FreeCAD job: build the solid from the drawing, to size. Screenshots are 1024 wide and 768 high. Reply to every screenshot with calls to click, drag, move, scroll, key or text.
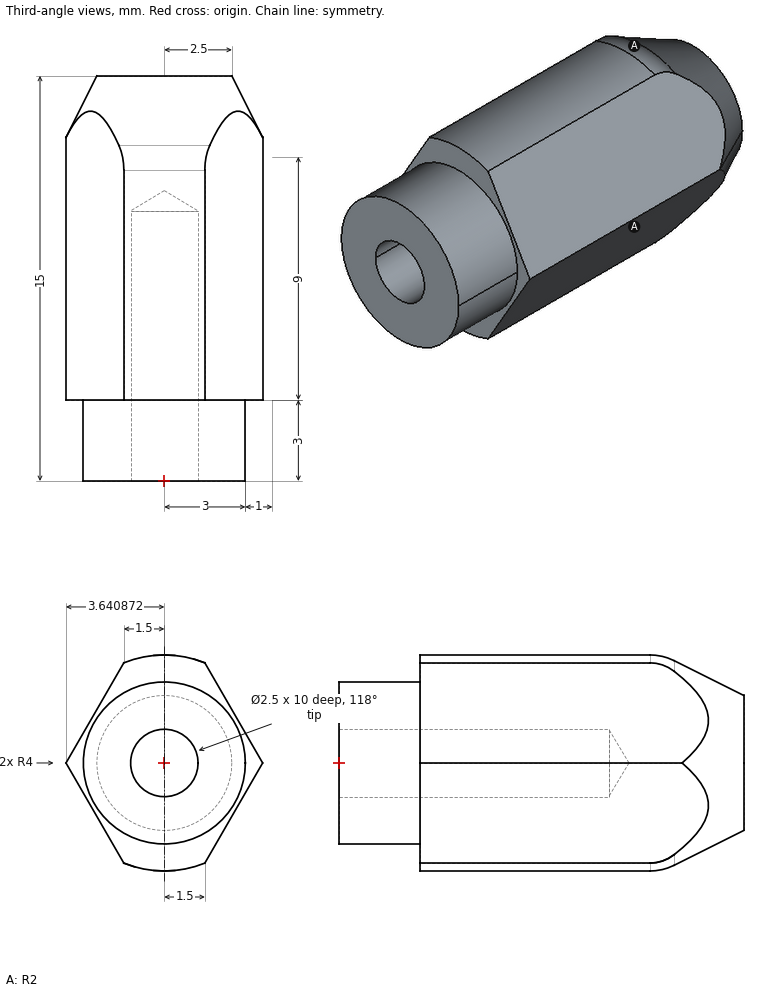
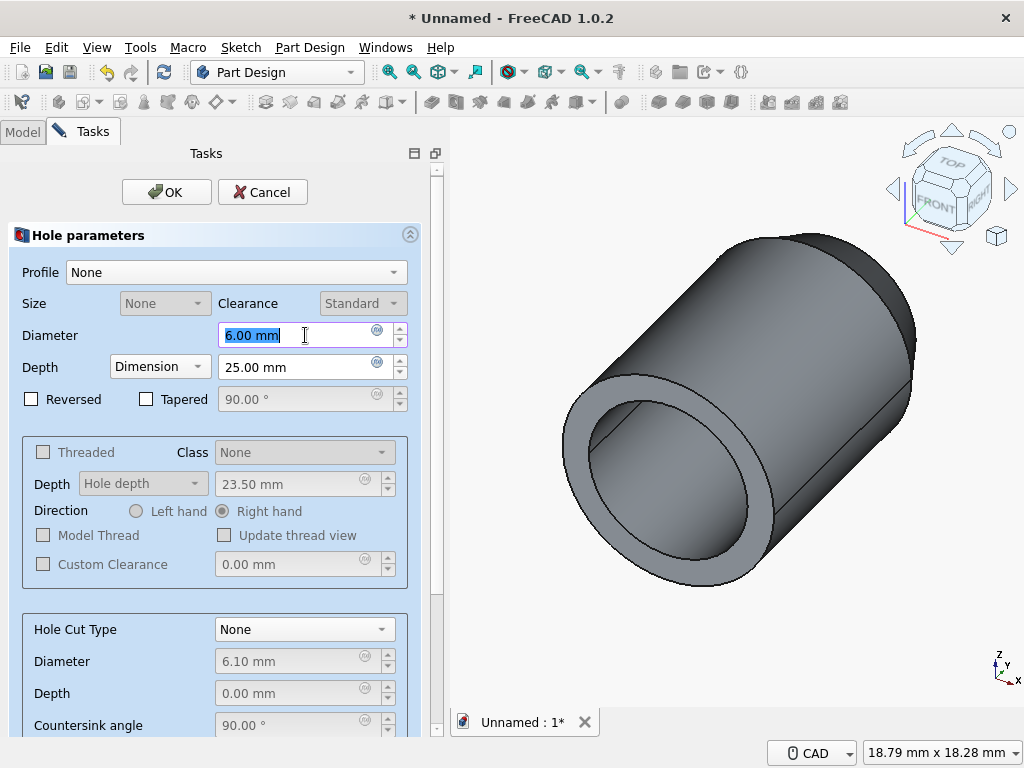
text(2.5)
key(Tab)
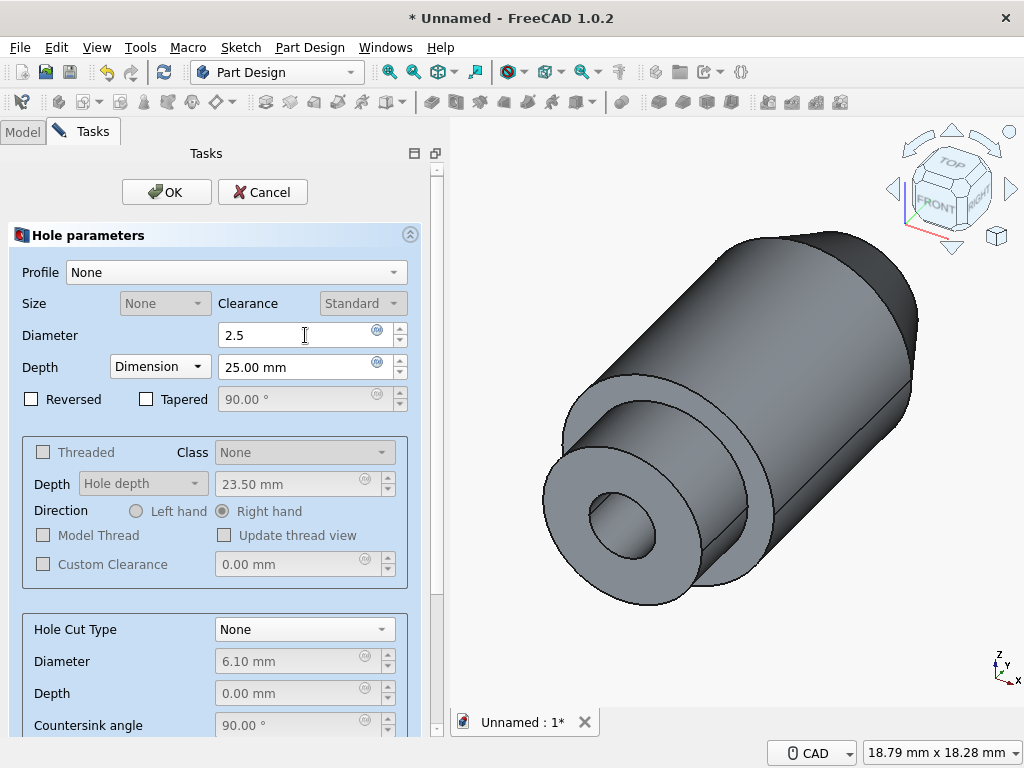
triple_click(305, 367)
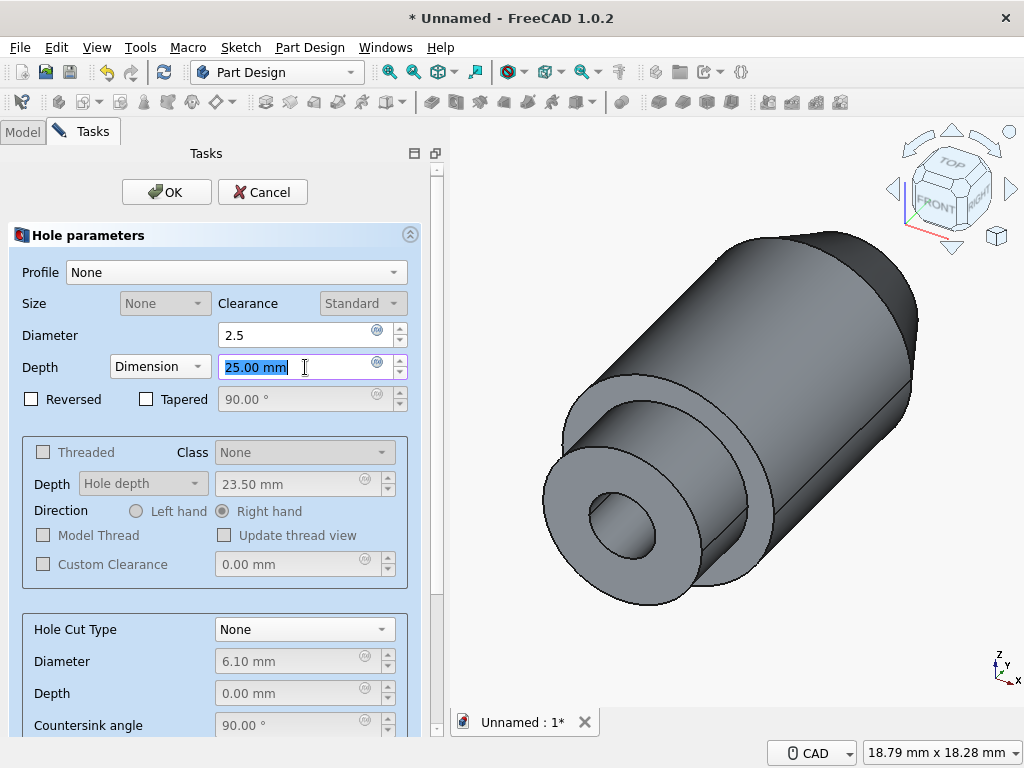
text(10)
key(Tab)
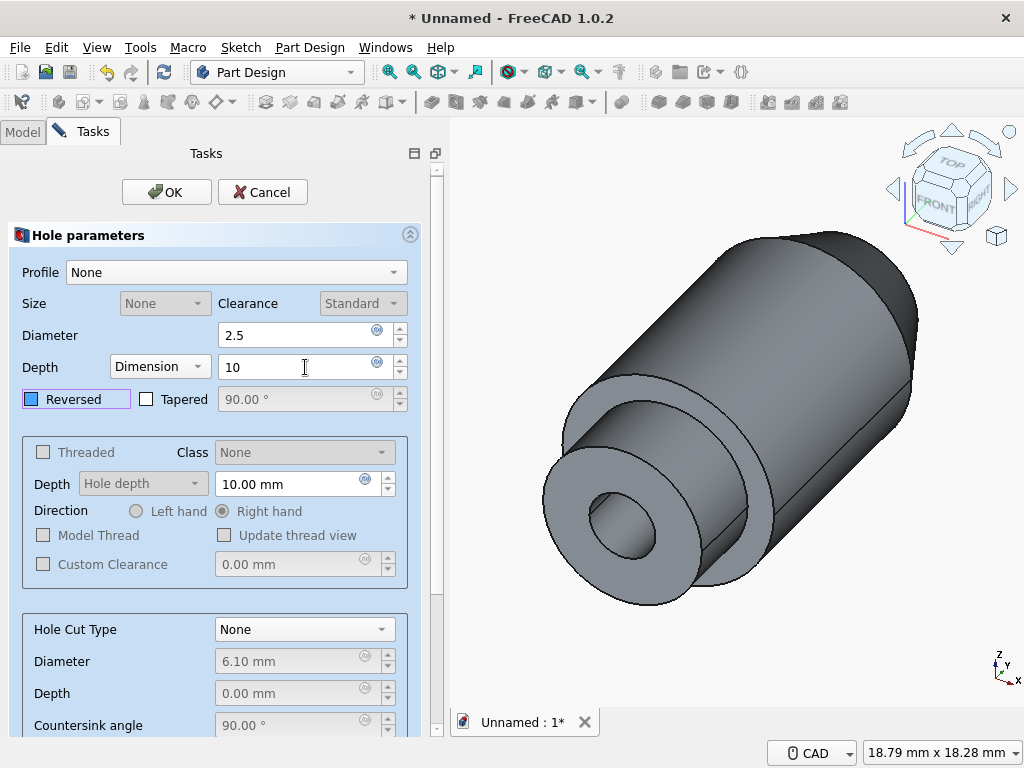
click(167, 192)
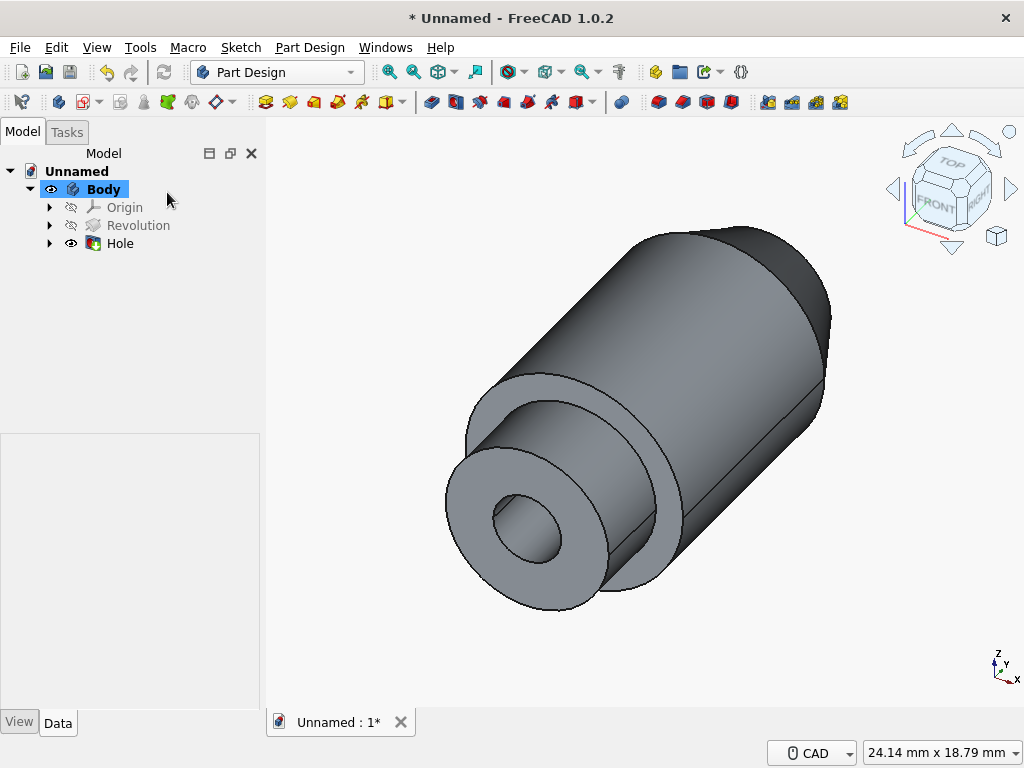
key(4)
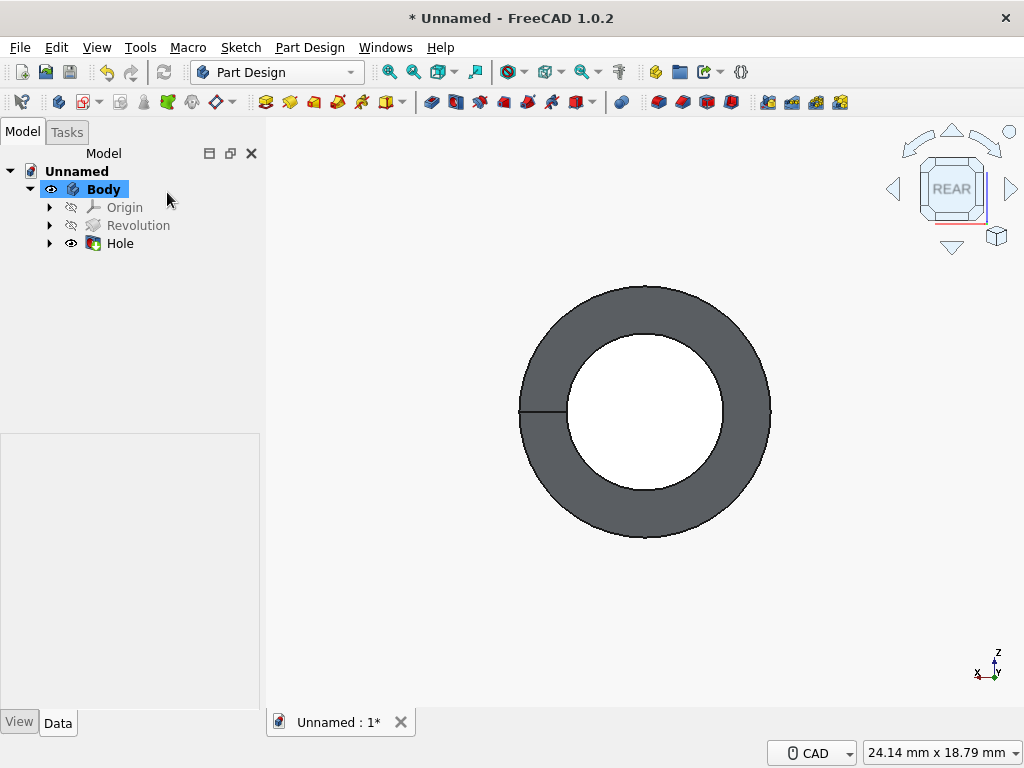
click(390, 72)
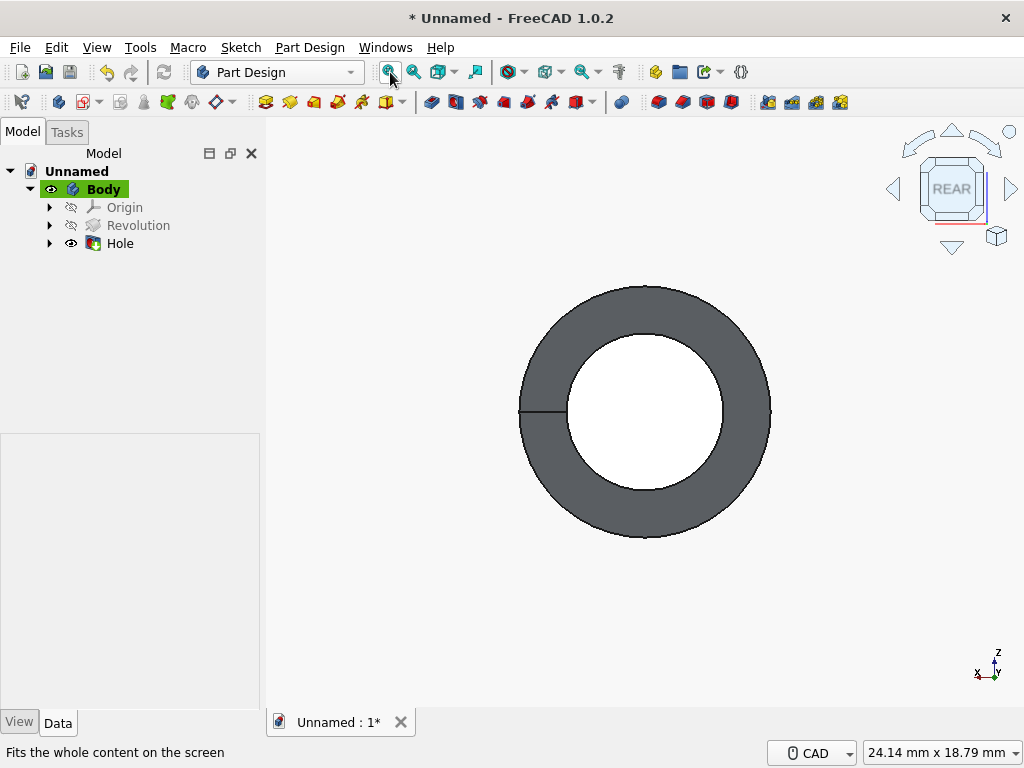
click(645, 411)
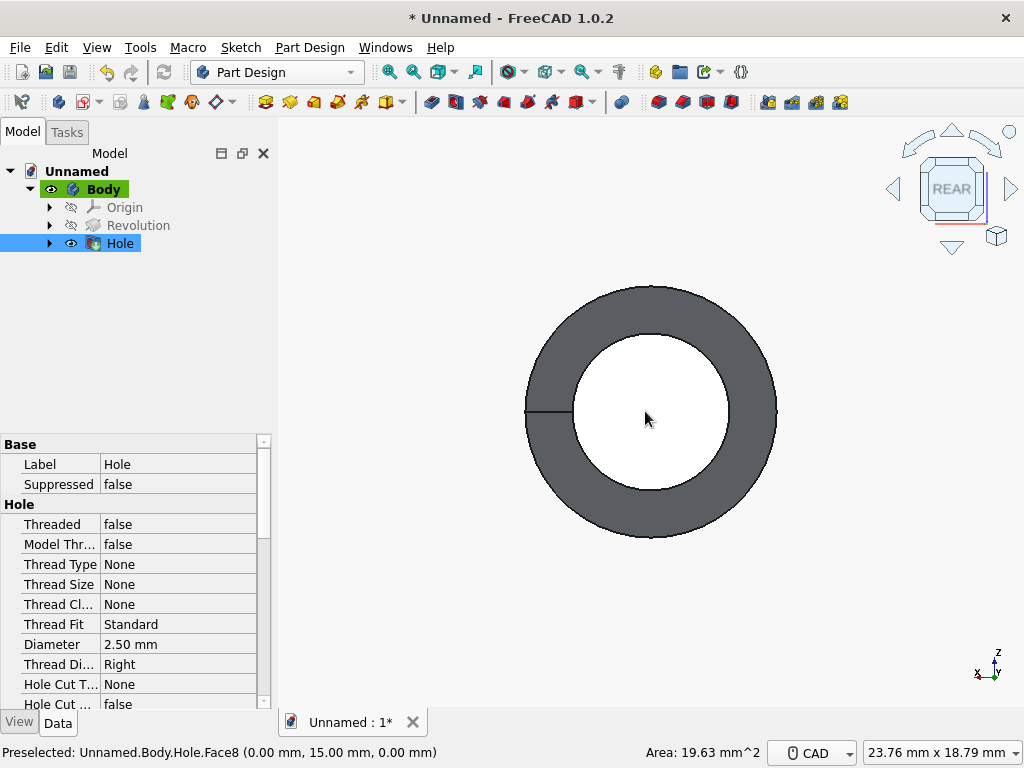
click(84, 102)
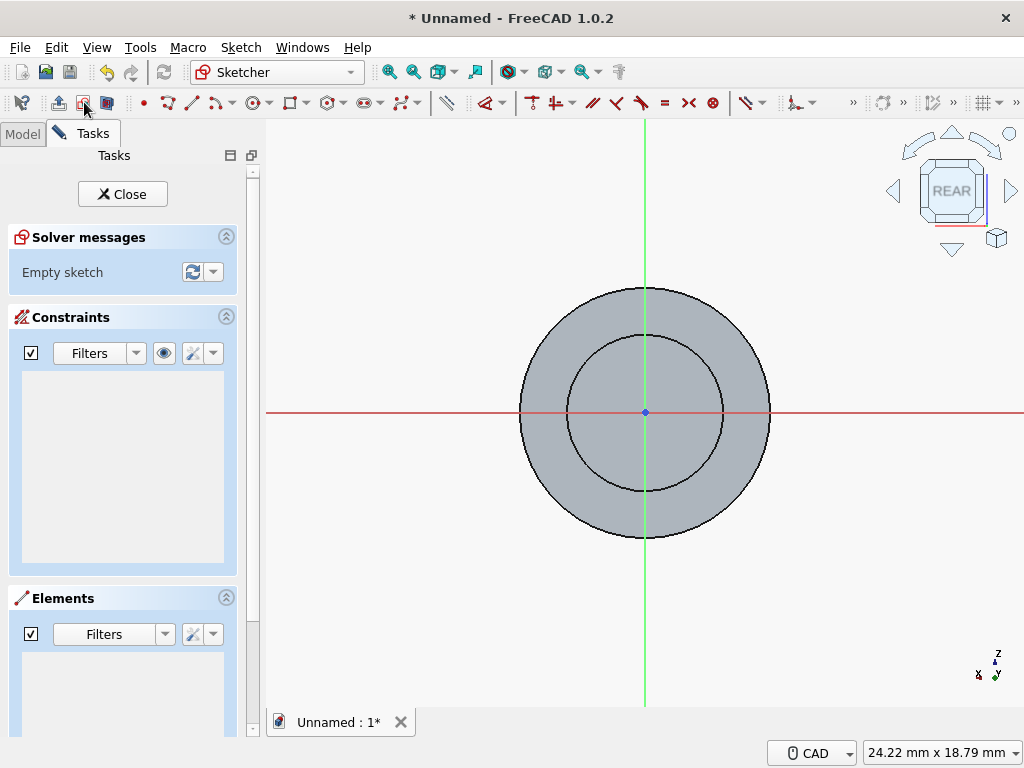
scroll(784, 413, up, 2)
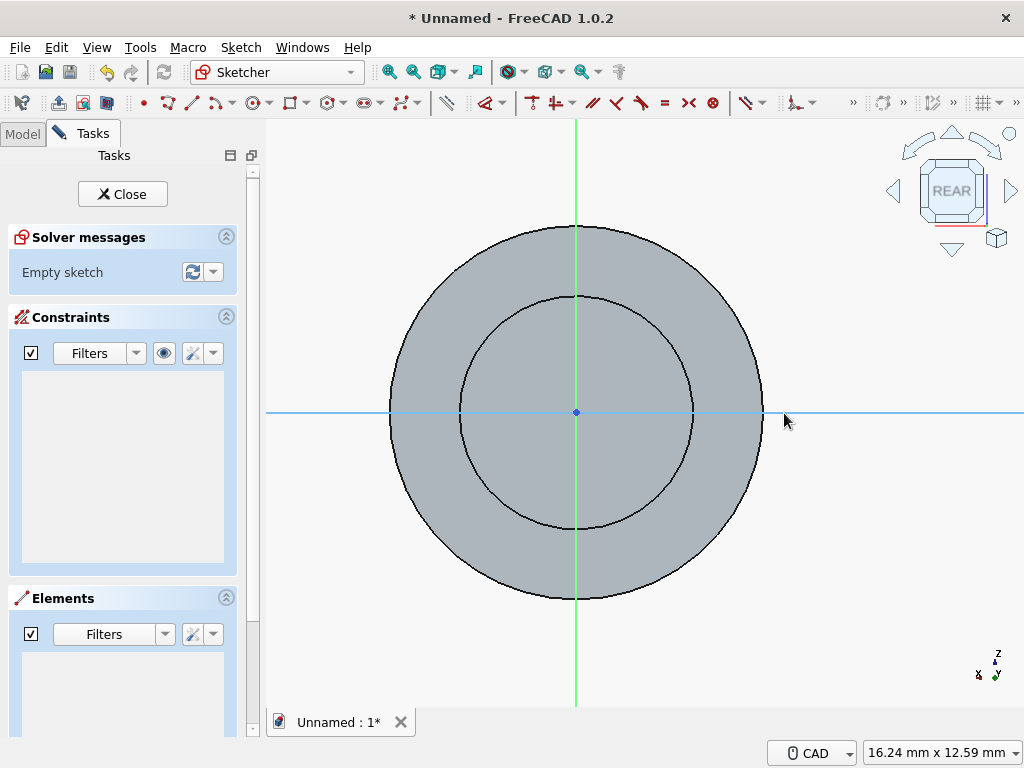
click(168, 104)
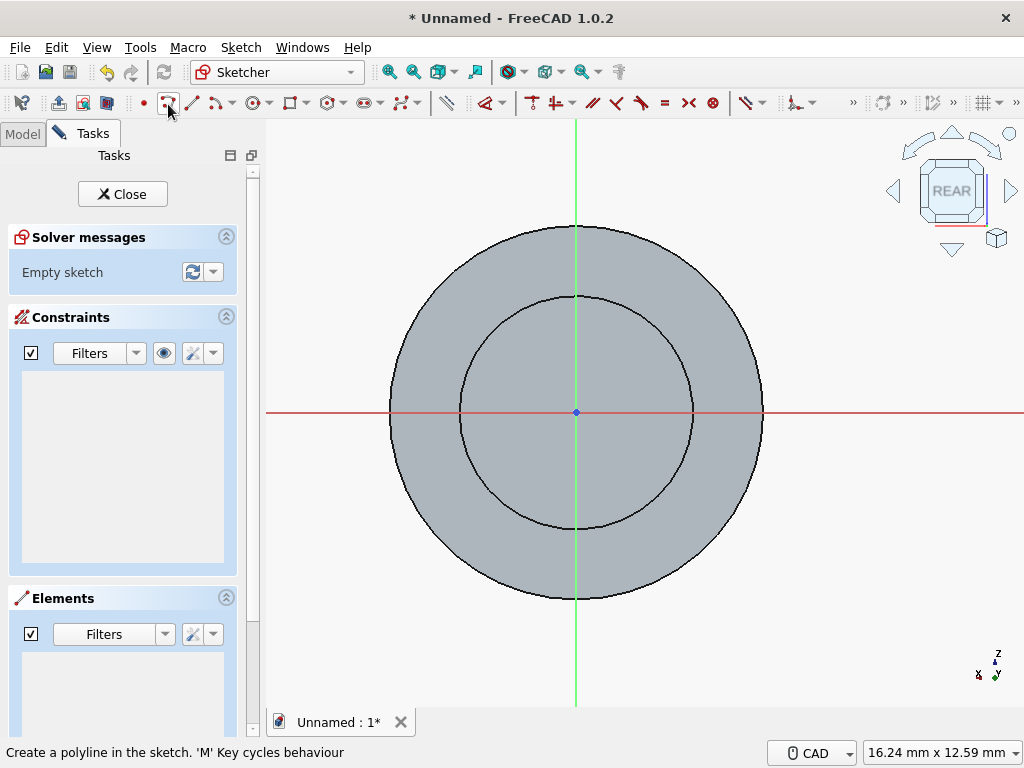
click(646, 240)
click(746, 413)
click(646, 586)
right_click(646, 586)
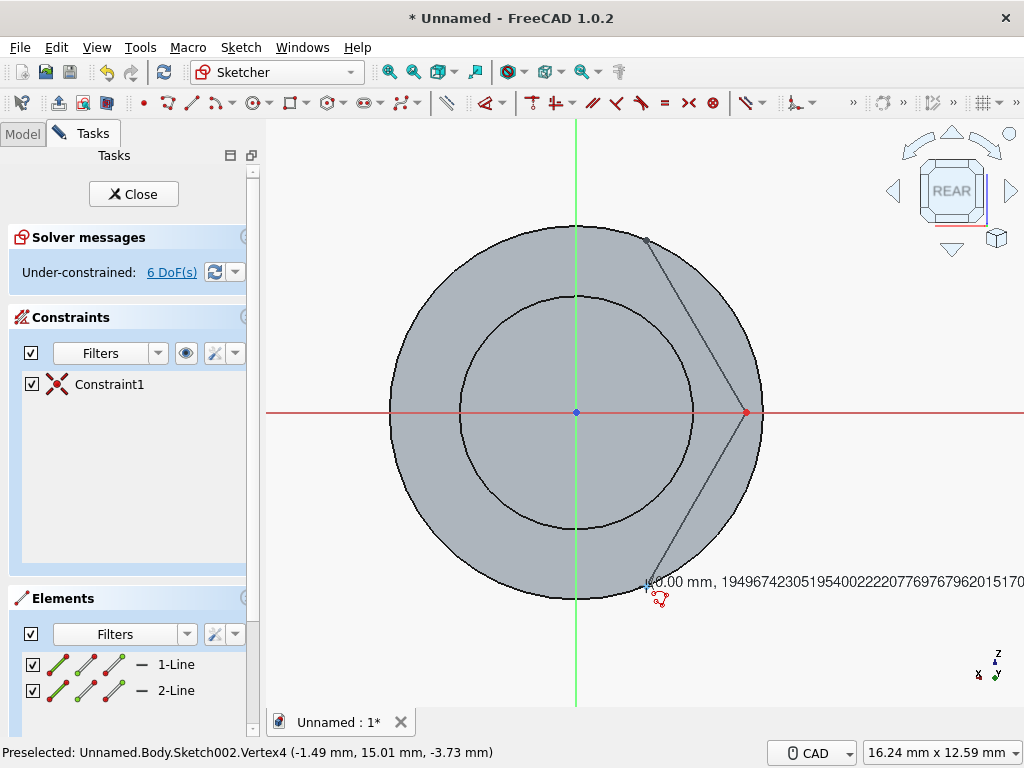
key(g)
key(3)
key(a)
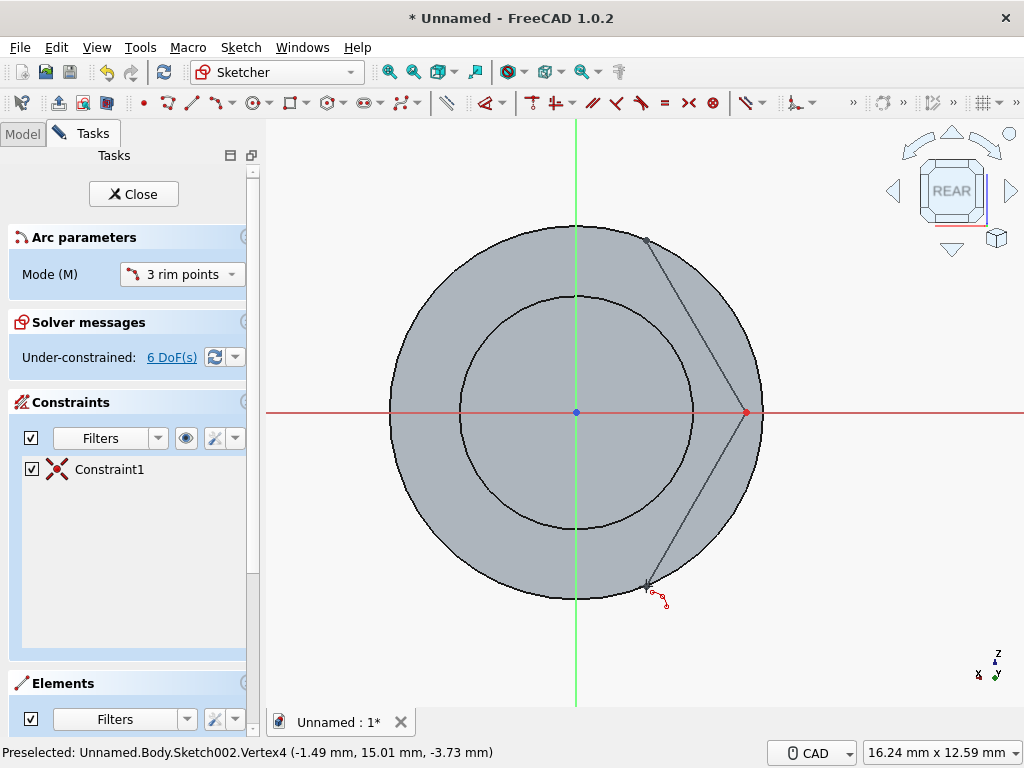
click(646, 587)
click(646, 241)
click(758, 457)